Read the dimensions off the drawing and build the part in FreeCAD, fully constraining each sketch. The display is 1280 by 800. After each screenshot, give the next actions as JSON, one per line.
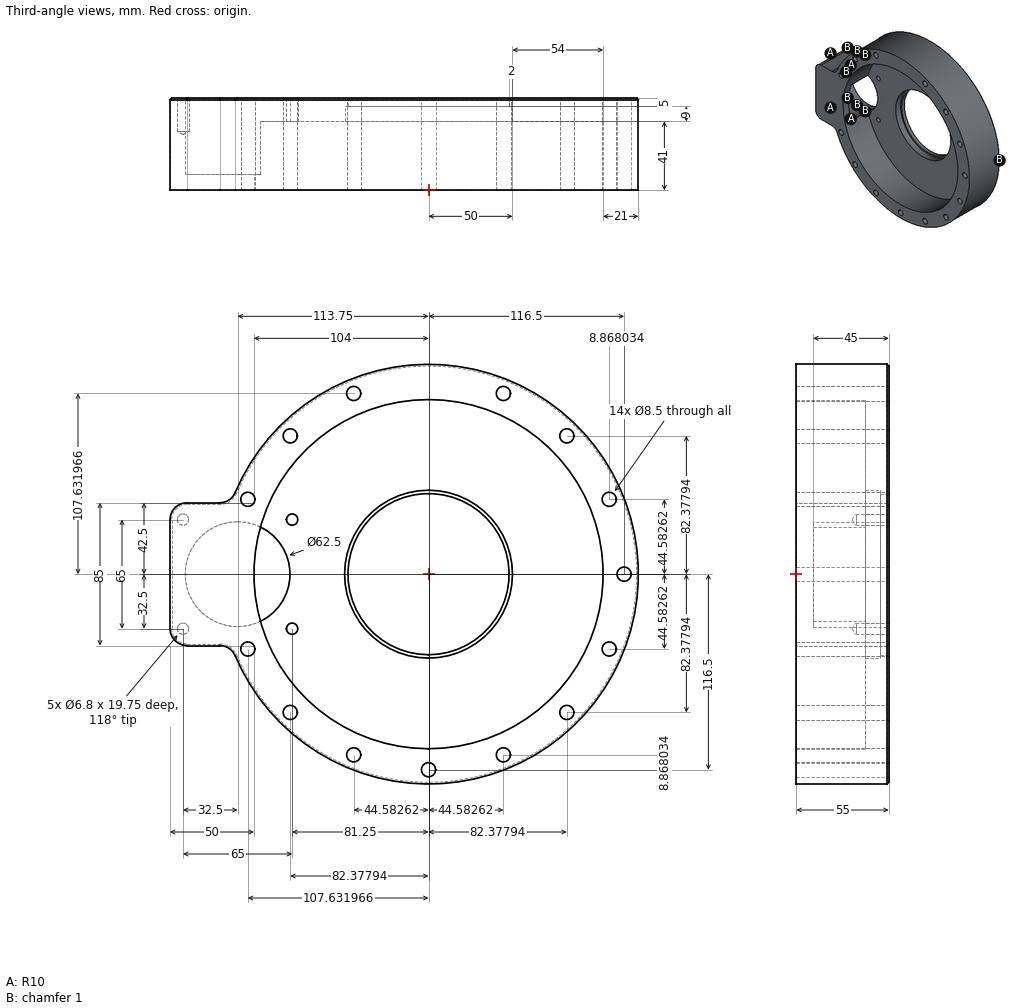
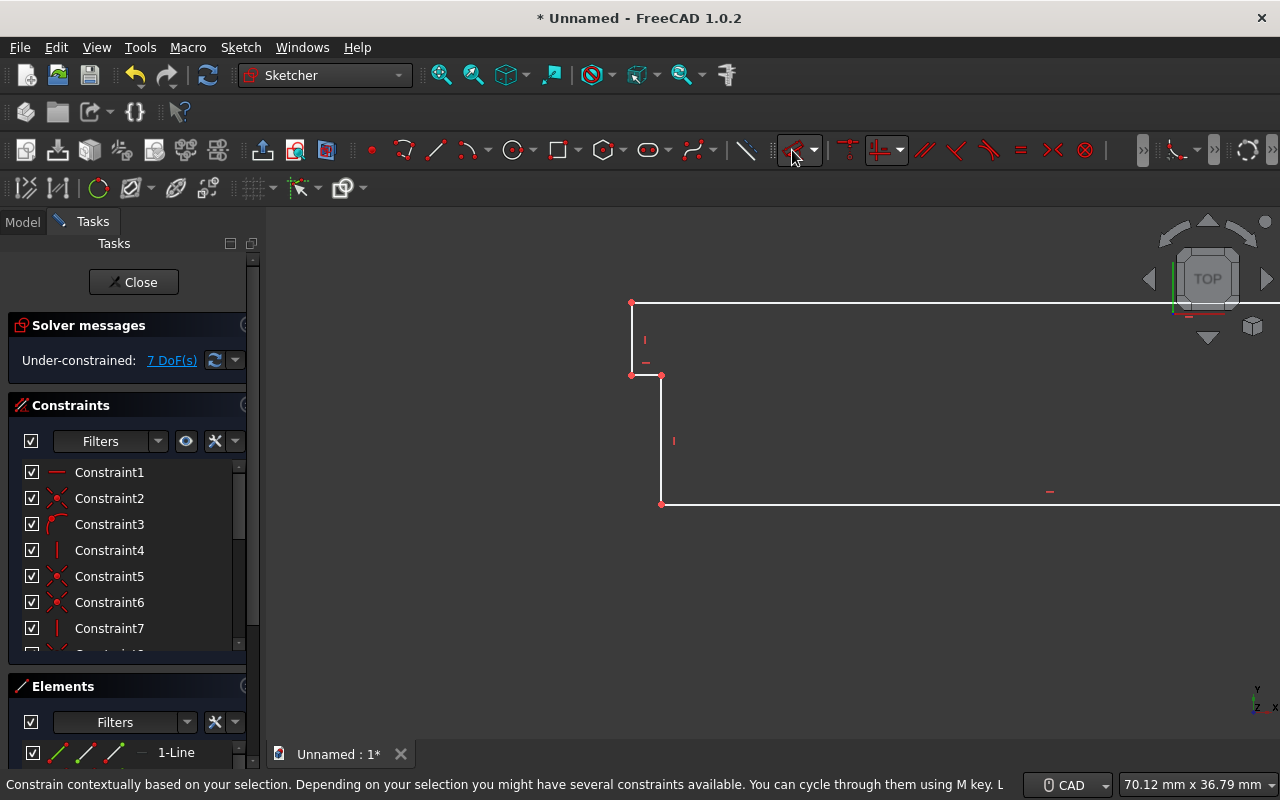
{"action": "left_click", "coordinate": [632, 325]}
{"action": "left_click", "coordinate": [598, 339]}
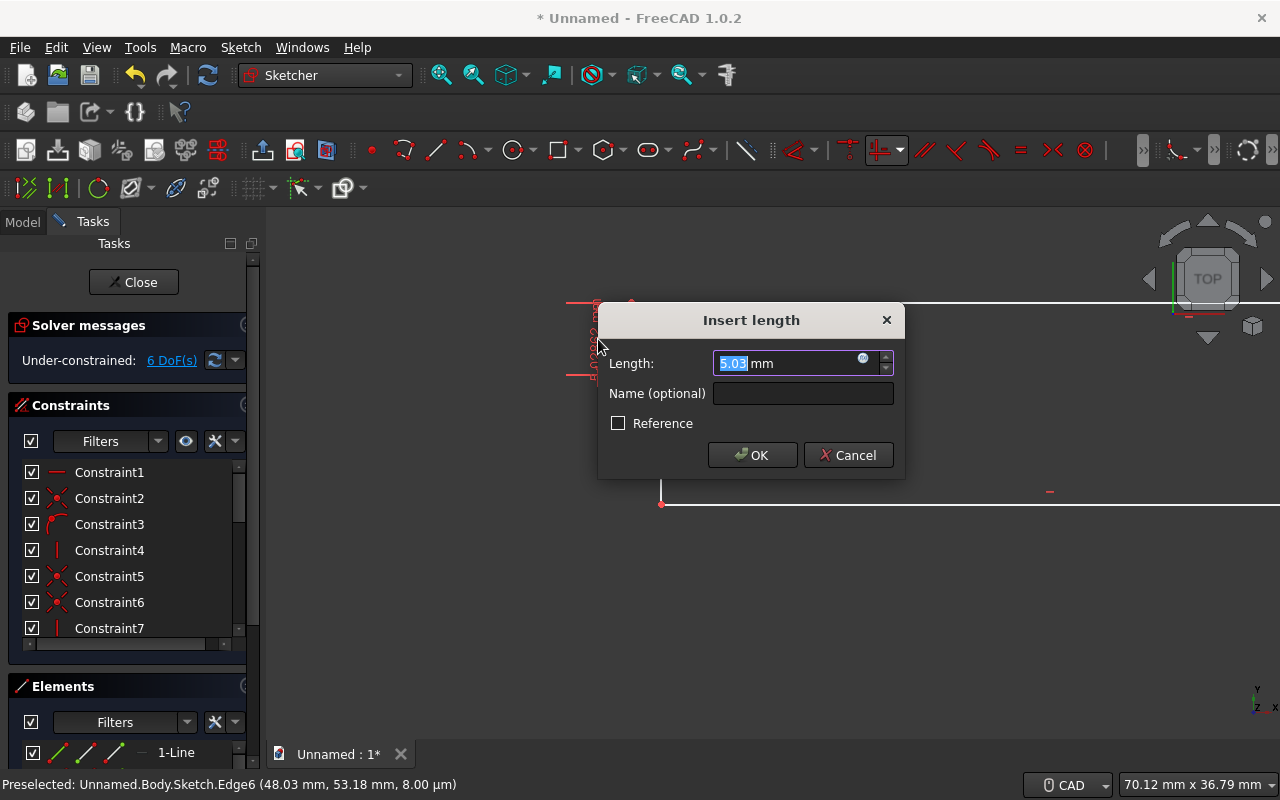
{"action": "type", "text": "5"}
{"action": "key", "text": "Return"}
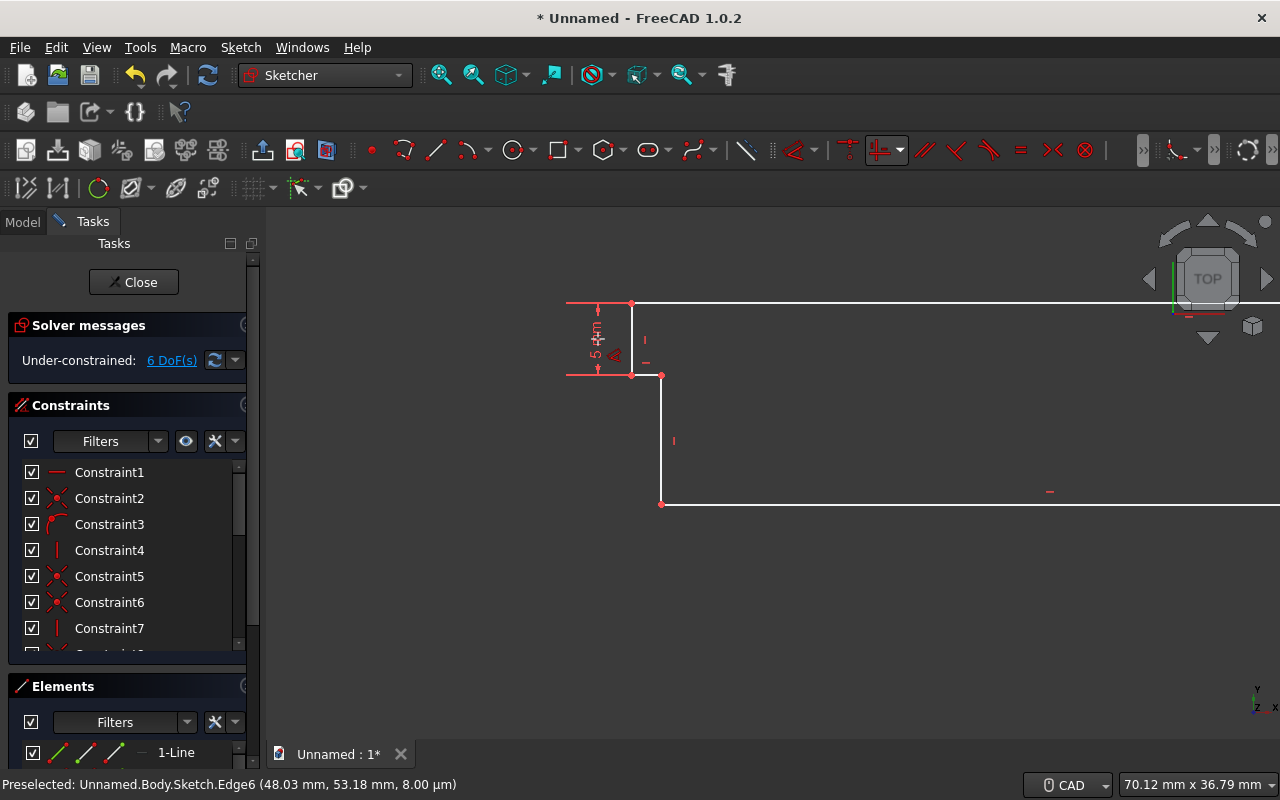
{"action": "scroll", "coordinate": [644, 375], "scroll_direction": "up", "scroll_amount": 2}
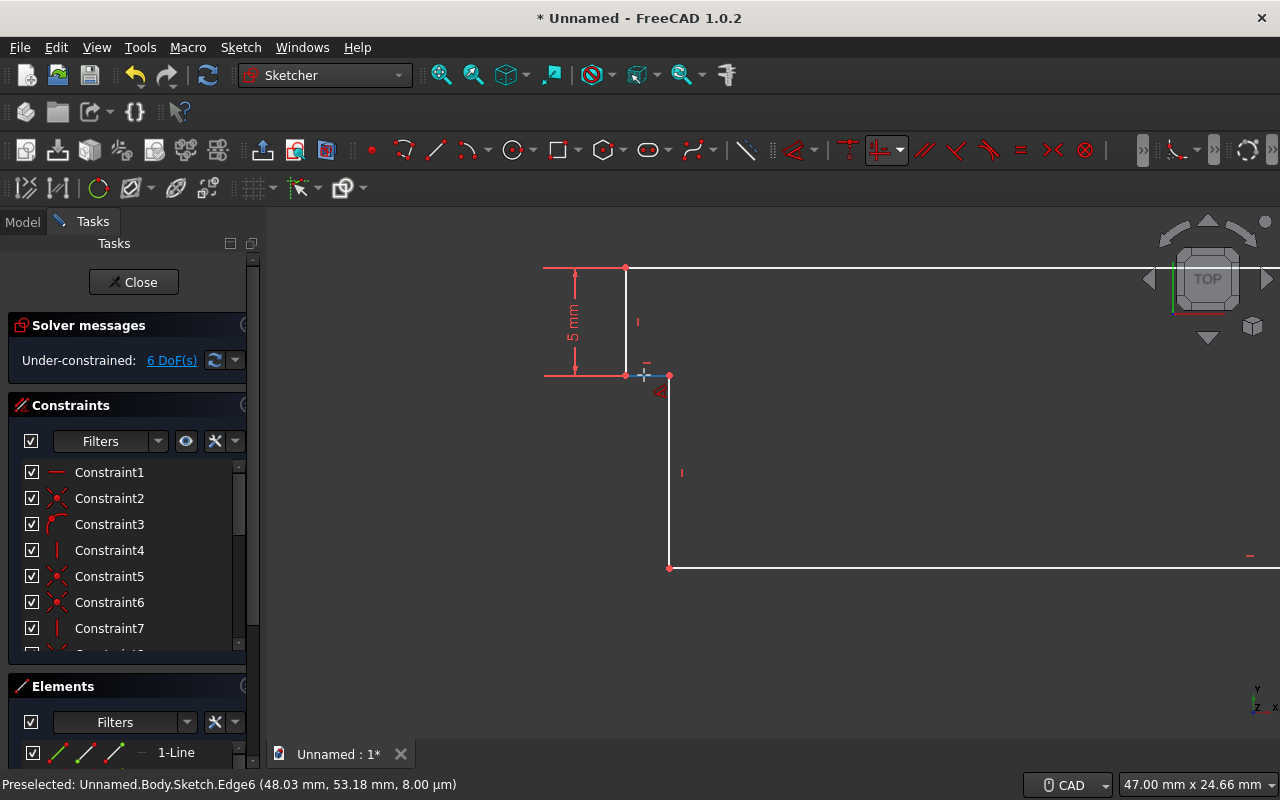
{"action": "left_click", "coordinate": [643, 376]}
{"action": "left_click", "coordinate": [648, 342]}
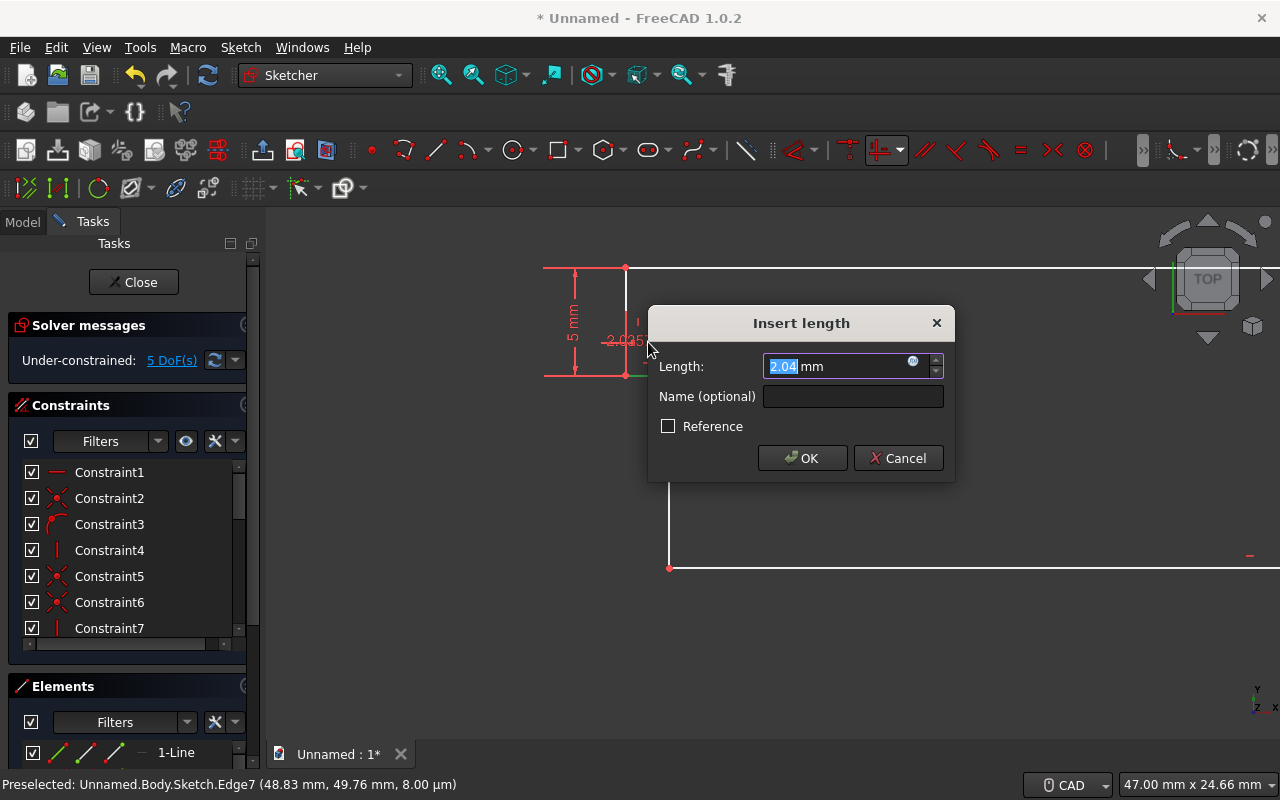
{"action": "type", "text": "2"}
{"action": "key", "text": "Return"}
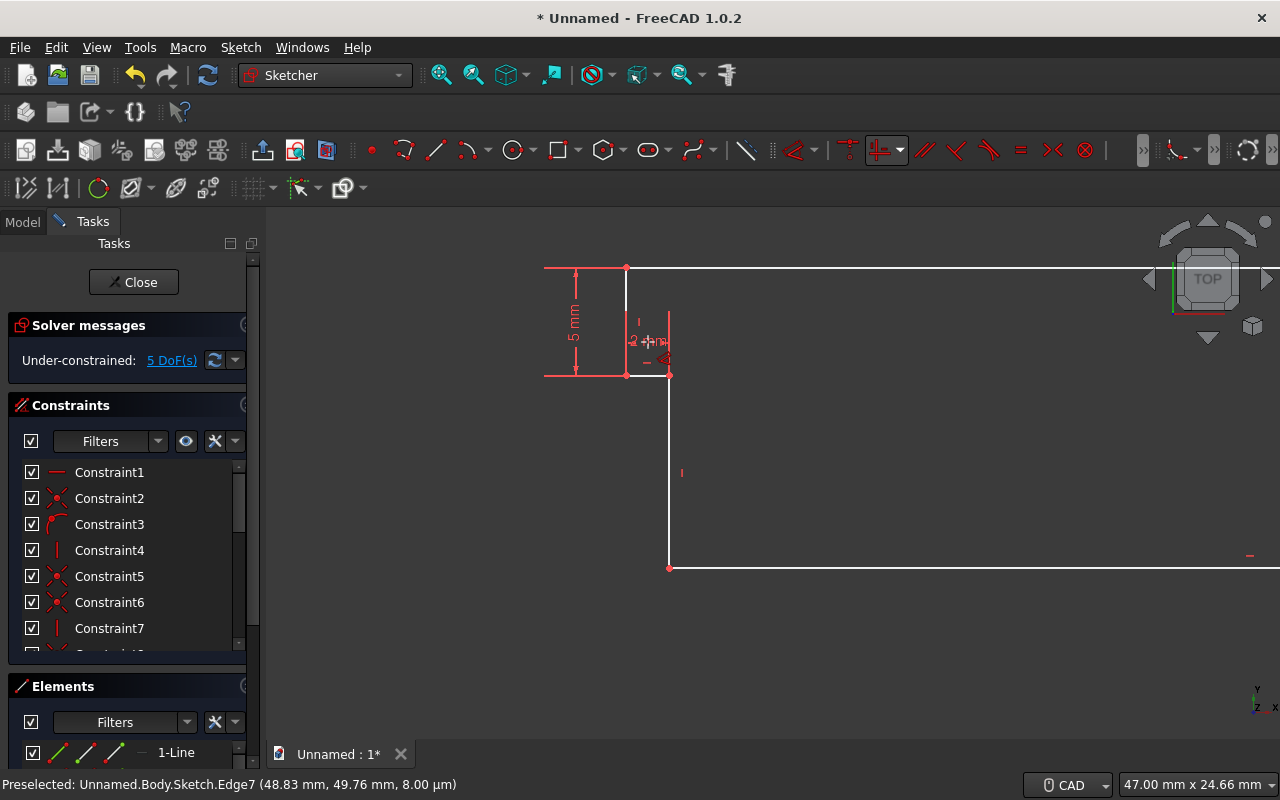
{"action": "scroll", "coordinate": [645, 376], "scroll_direction": "down", "scroll_amount": 8}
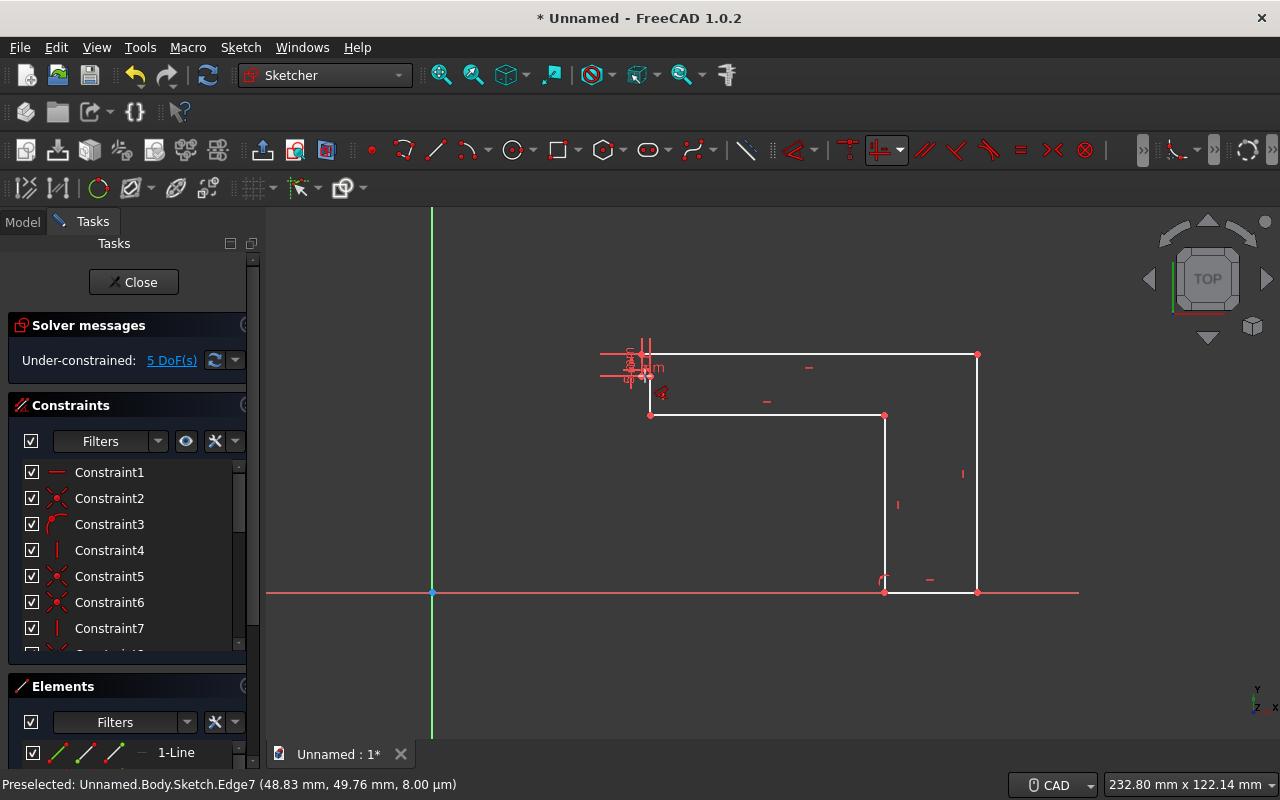
{"action": "left_click", "coordinate": [650, 388]}
{"action": "left_click", "coordinate": [616, 396]}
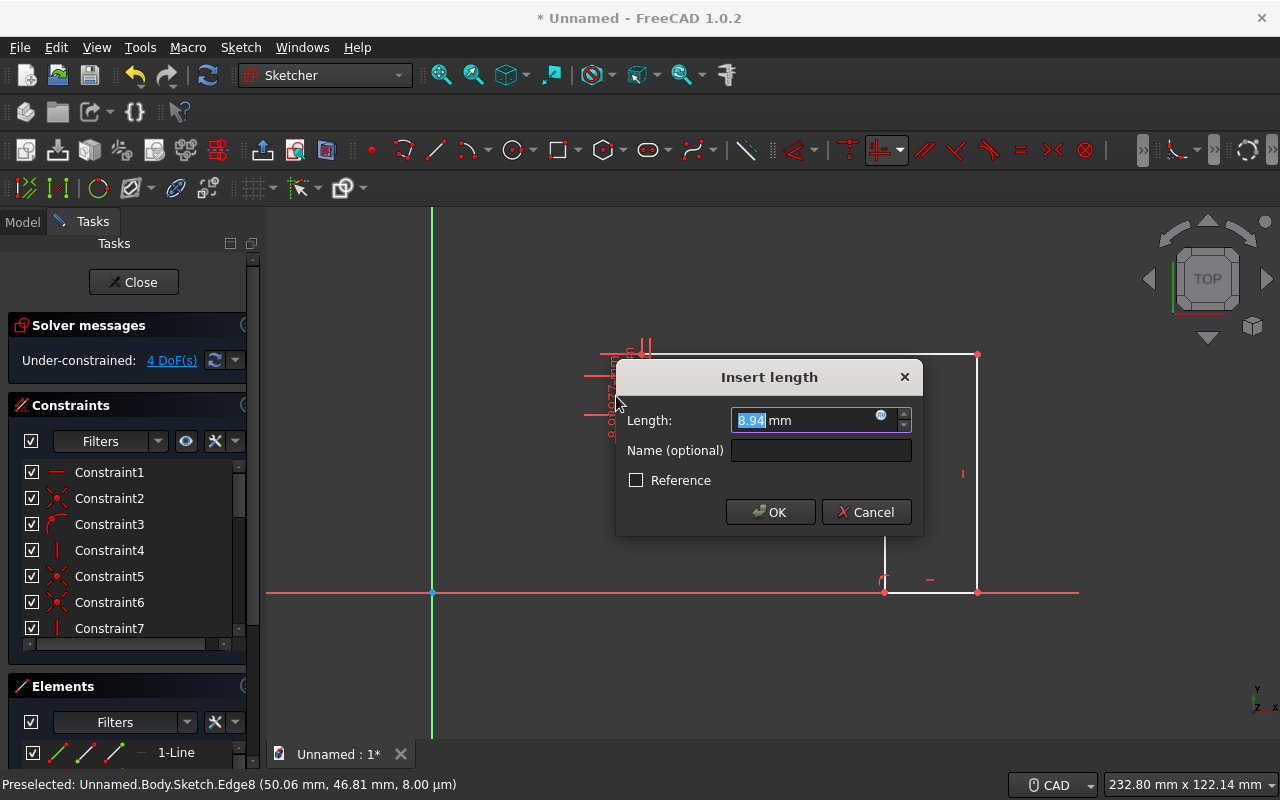
{"action": "type", "text": "9"}
{"action": "key", "text": "Return"}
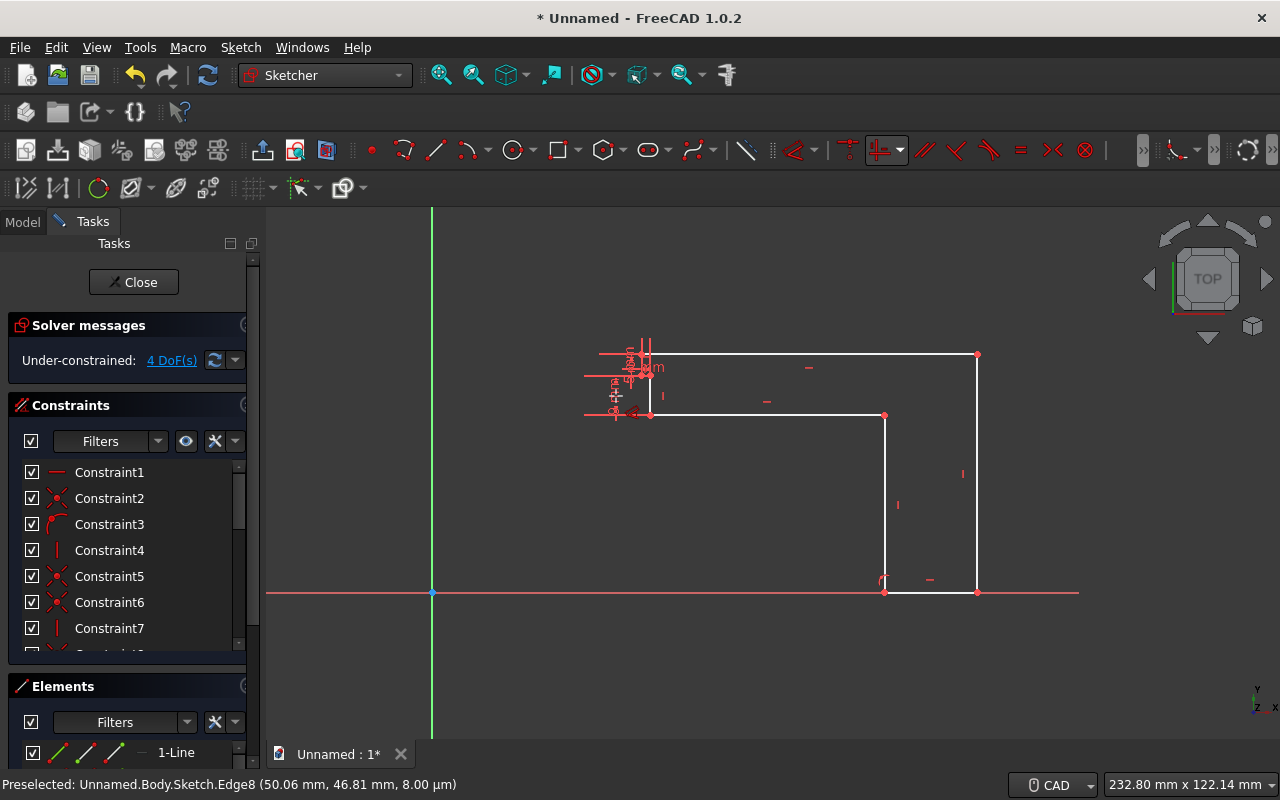
{"action": "left_click", "coordinate": [721, 415]}
{"action": "left_click", "coordinate": [767, 381]}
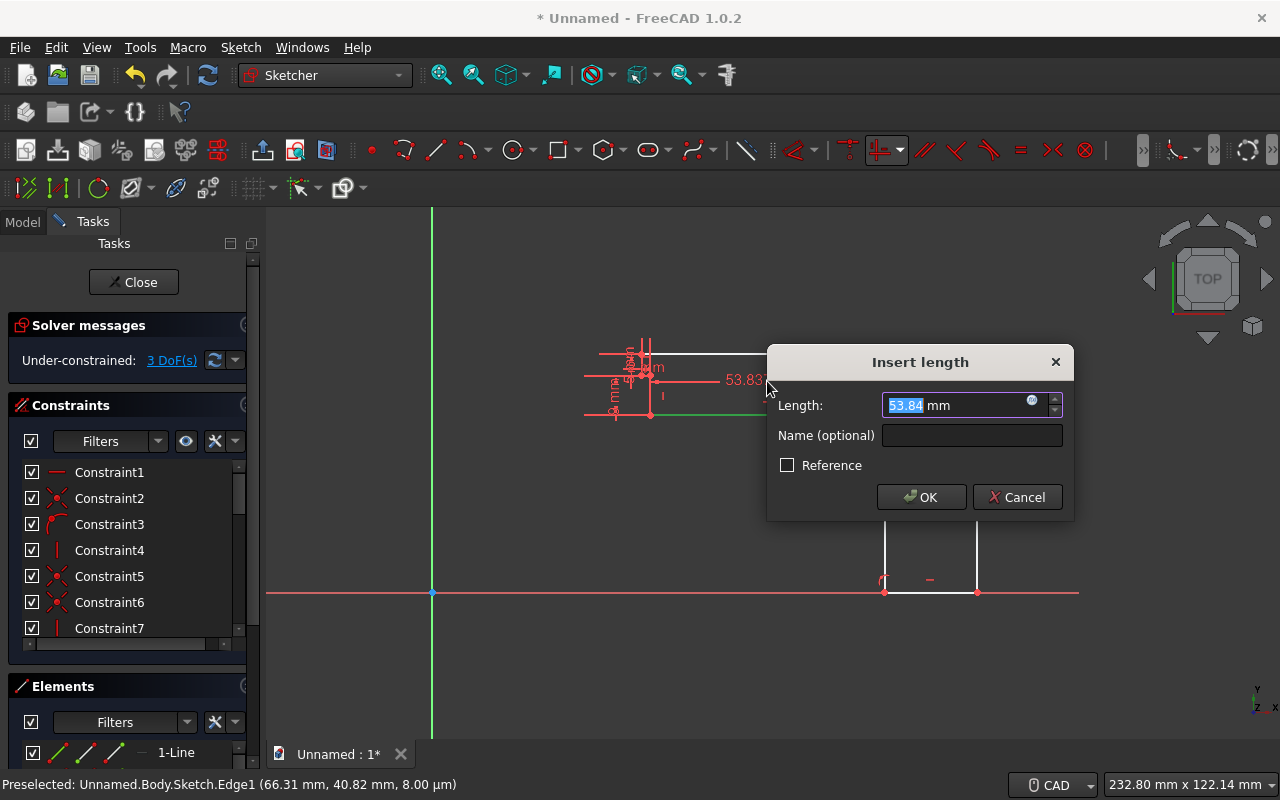
{"action": "type", "text": "54"}
{"action": "key", "text": "Return"}